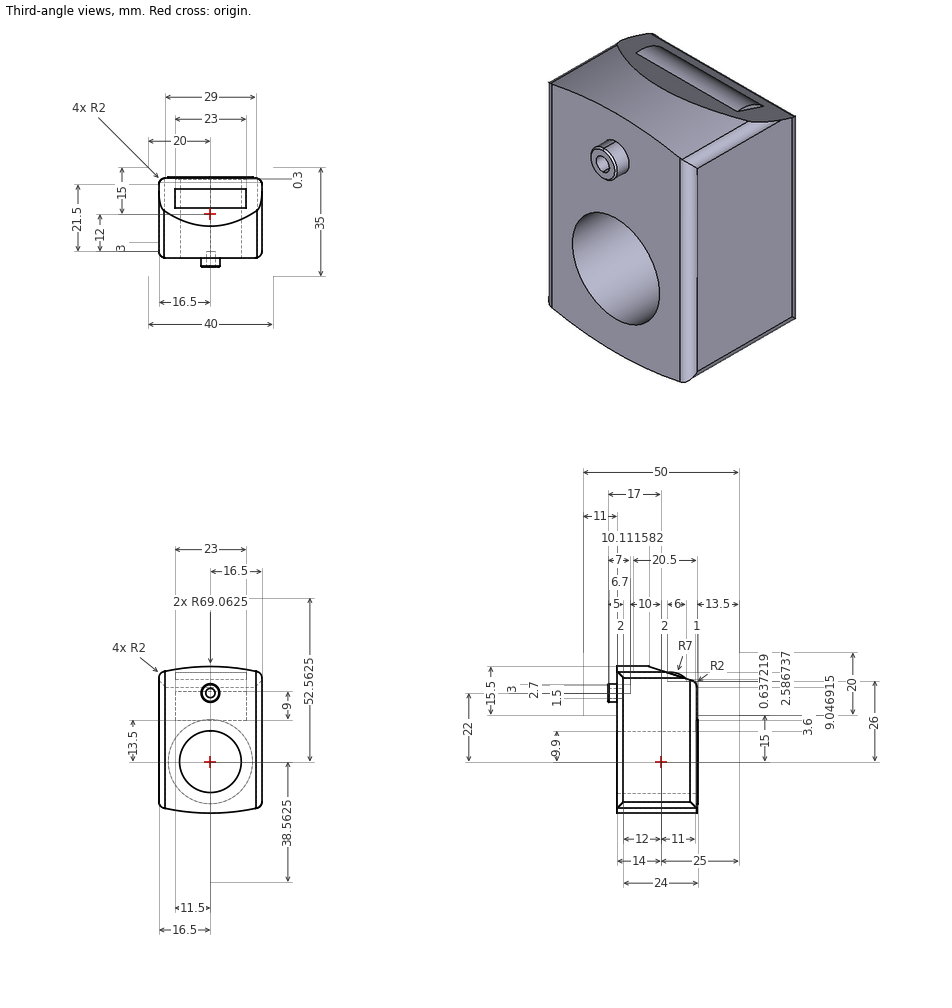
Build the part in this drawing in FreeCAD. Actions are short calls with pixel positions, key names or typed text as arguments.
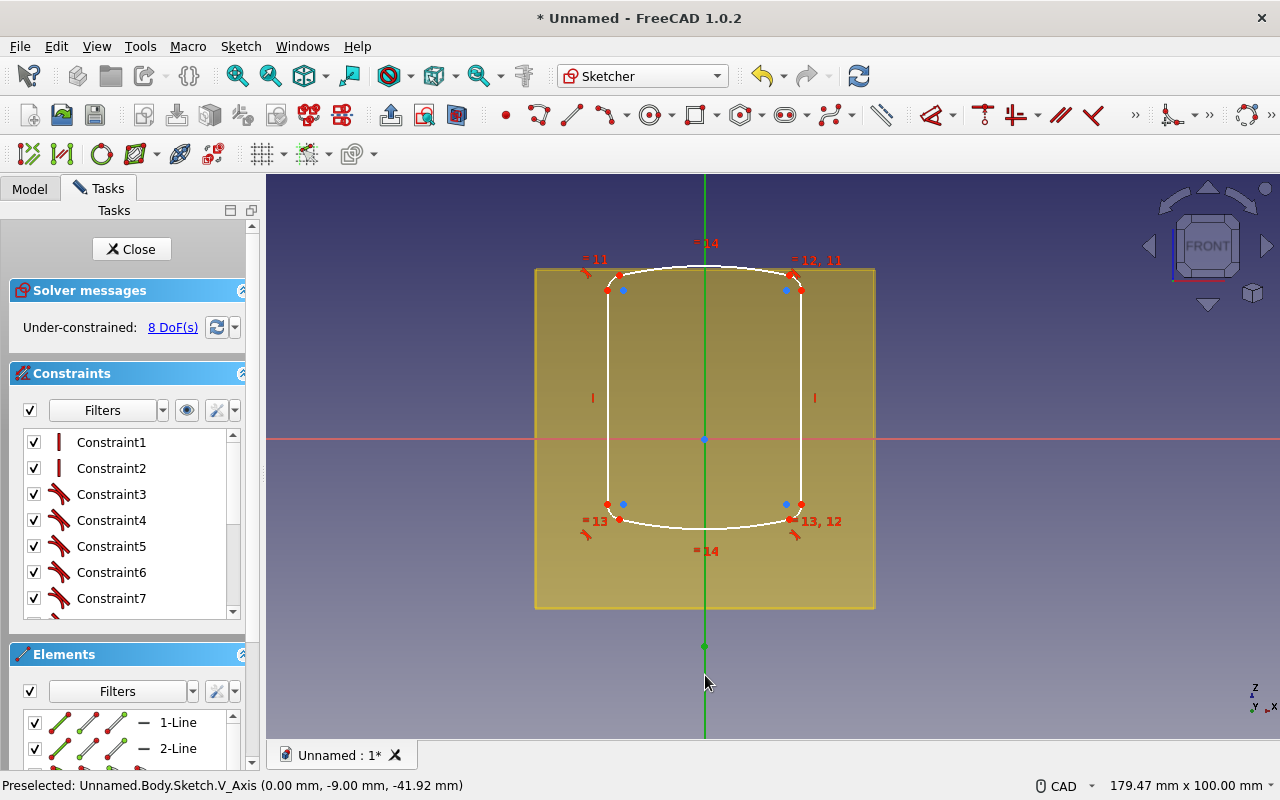
click(983, 116)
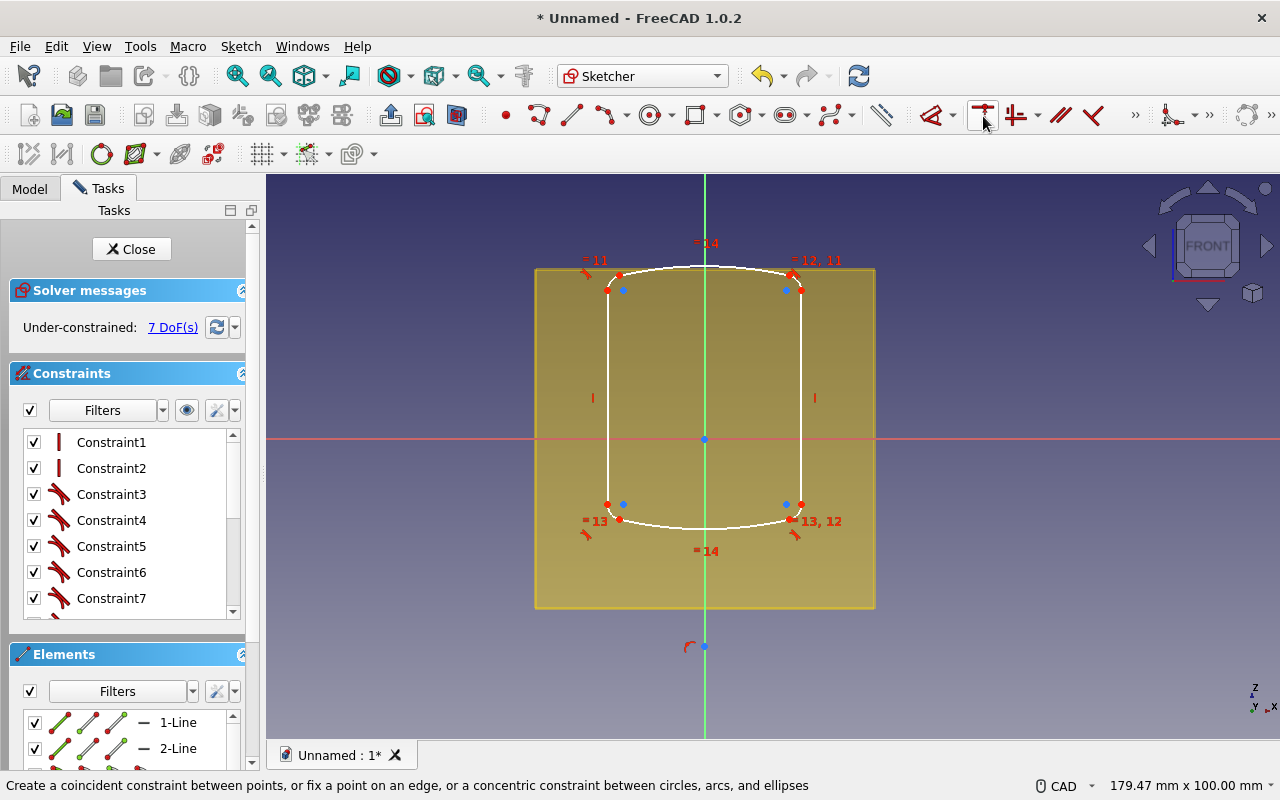
scroll(705, 284, up, 2)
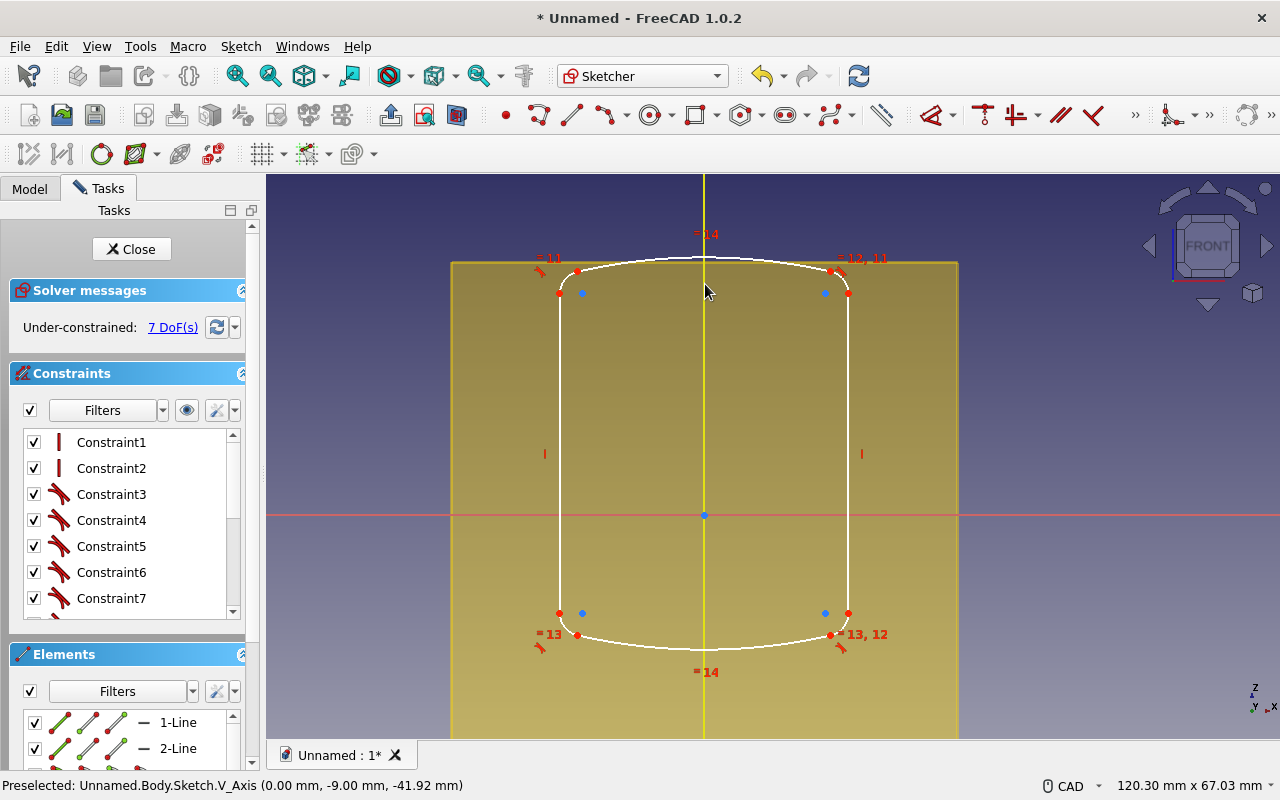
scroll(705, 635, down, 2)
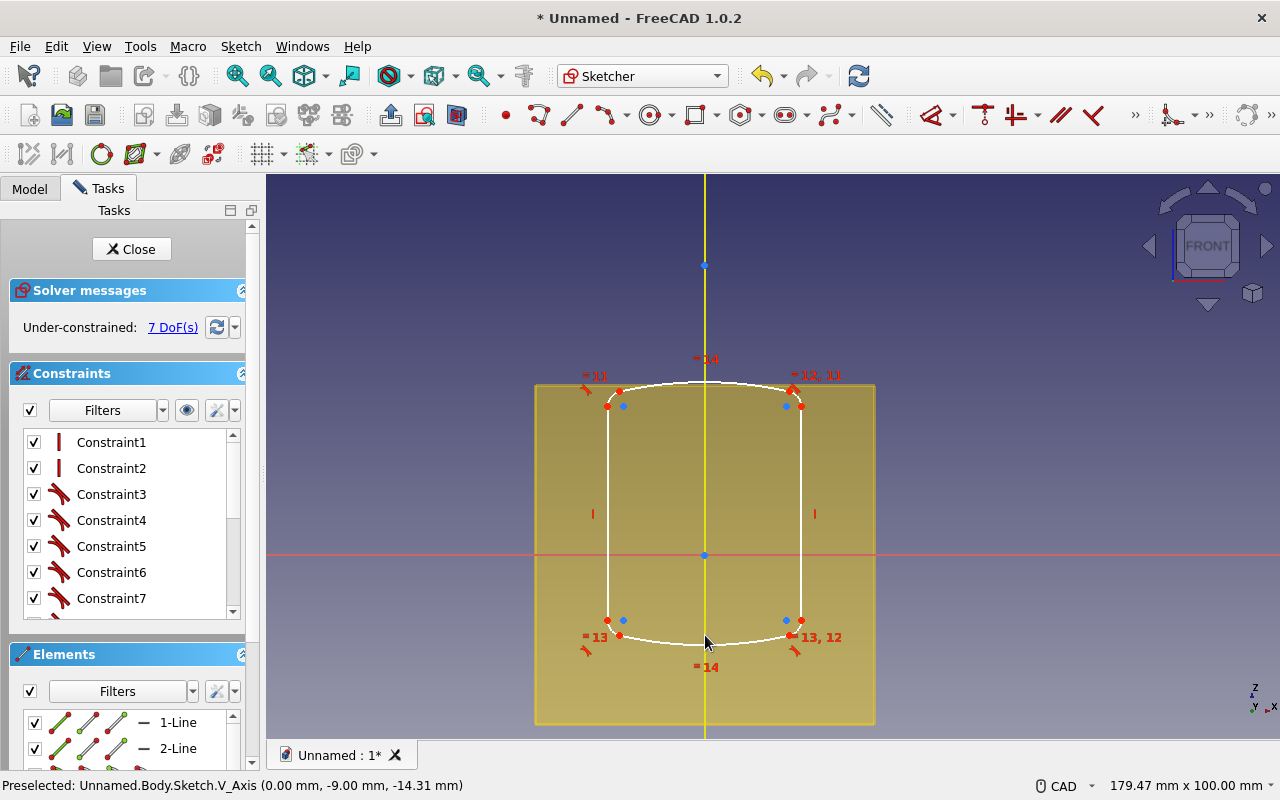
click(705, 265)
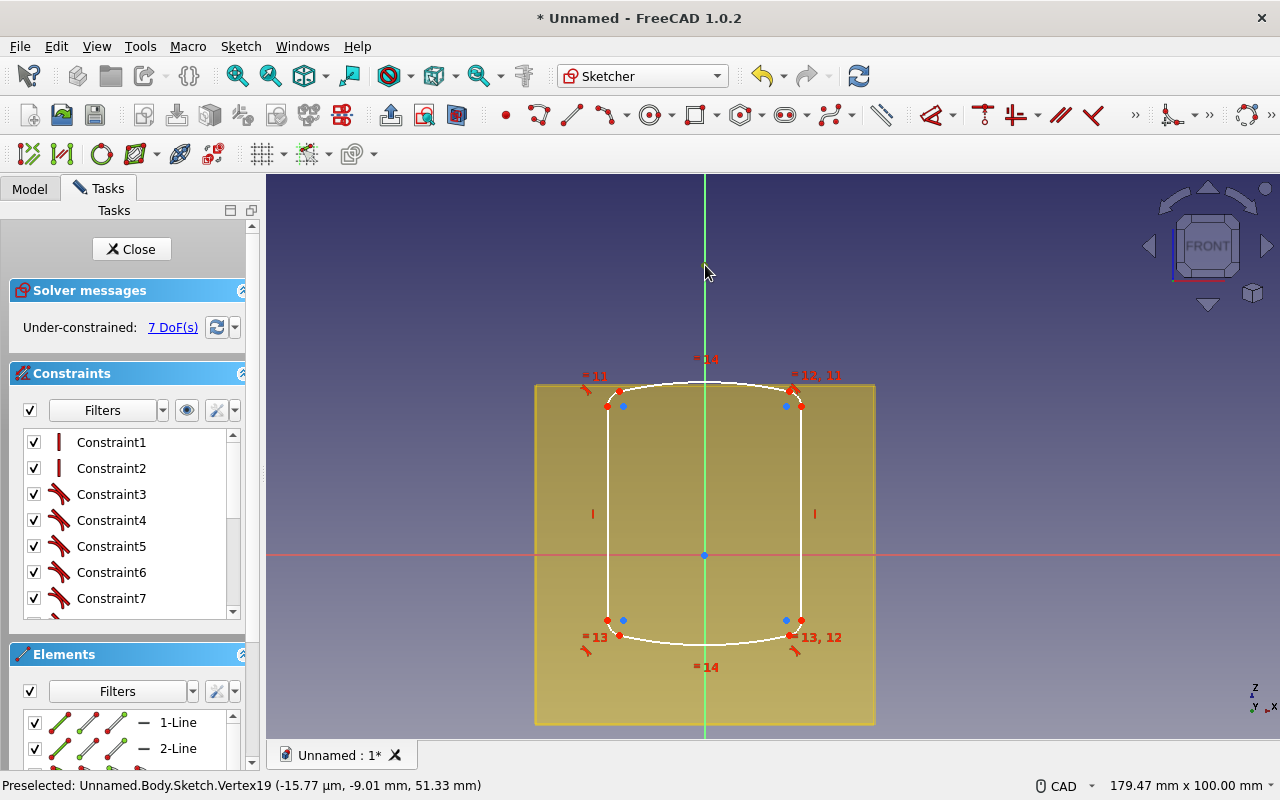
click(705, 602)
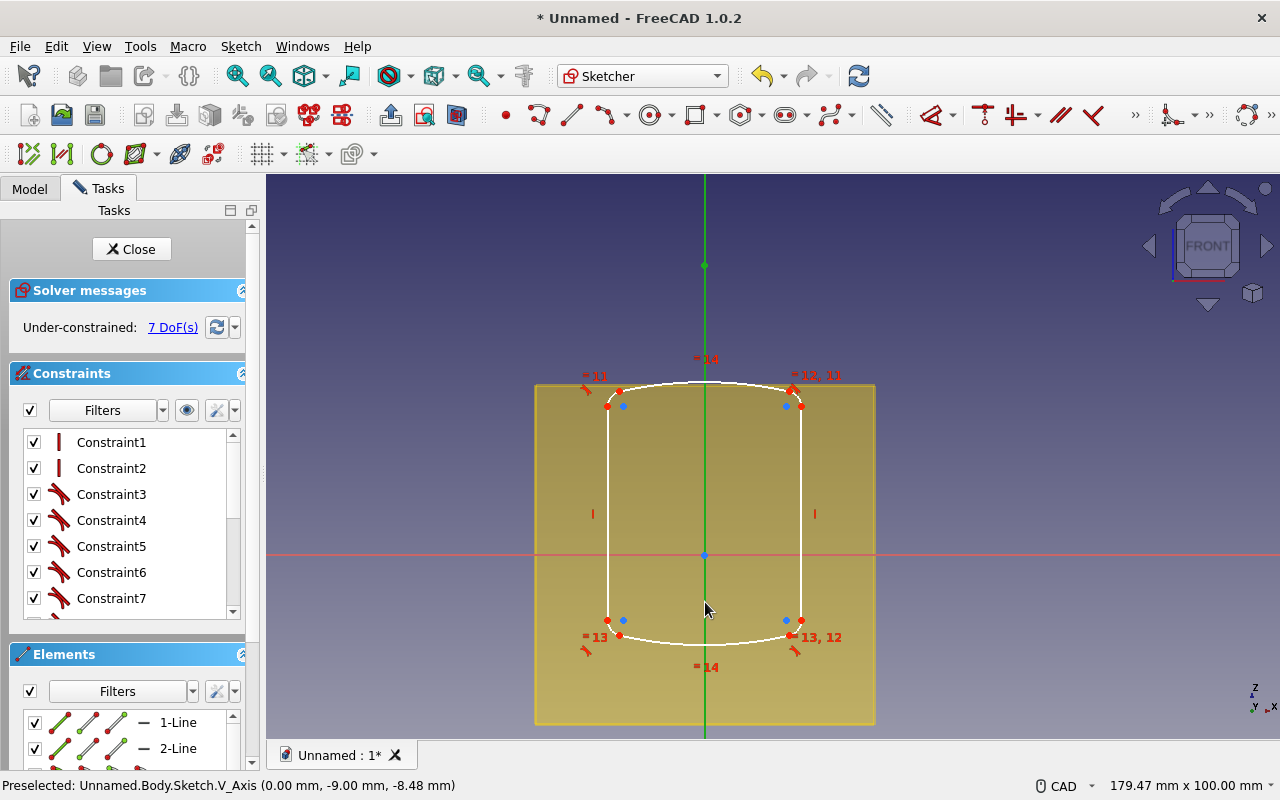
click(983, 116)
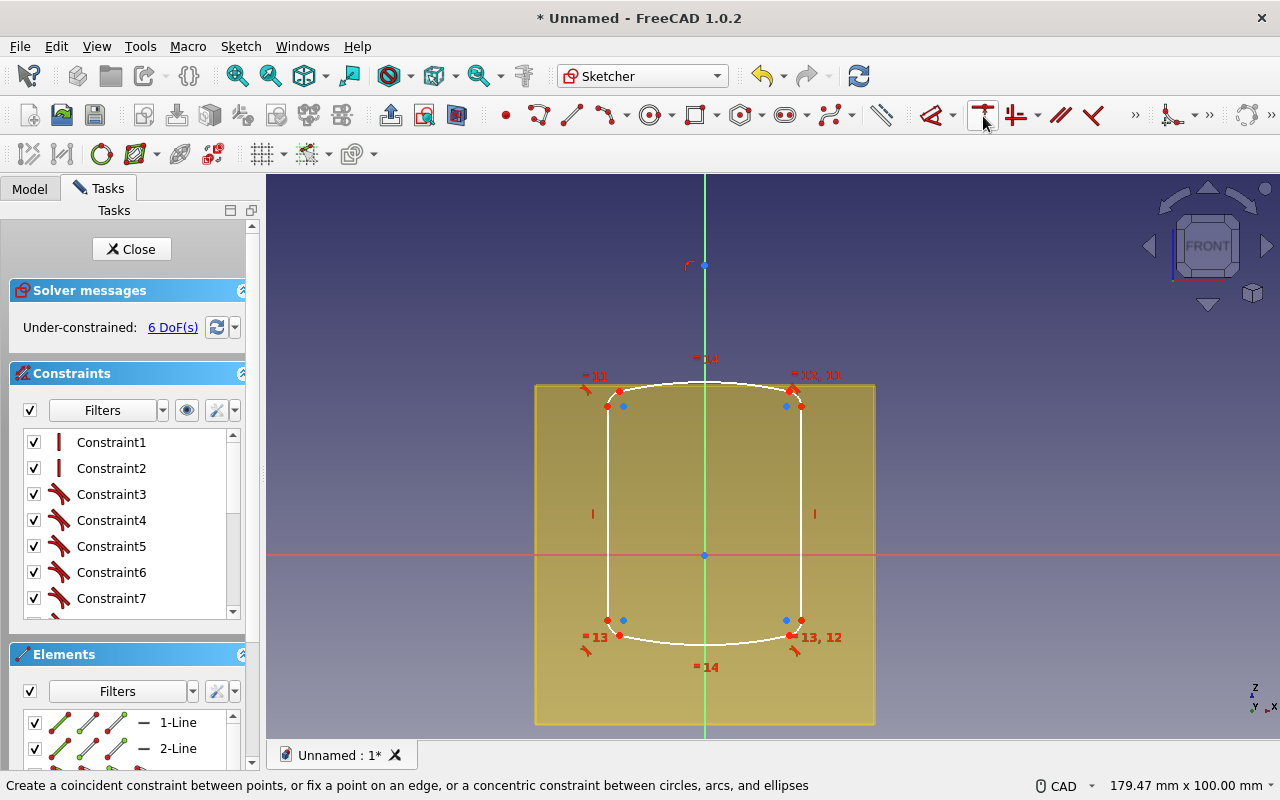
scroll(611, 397, up, 7)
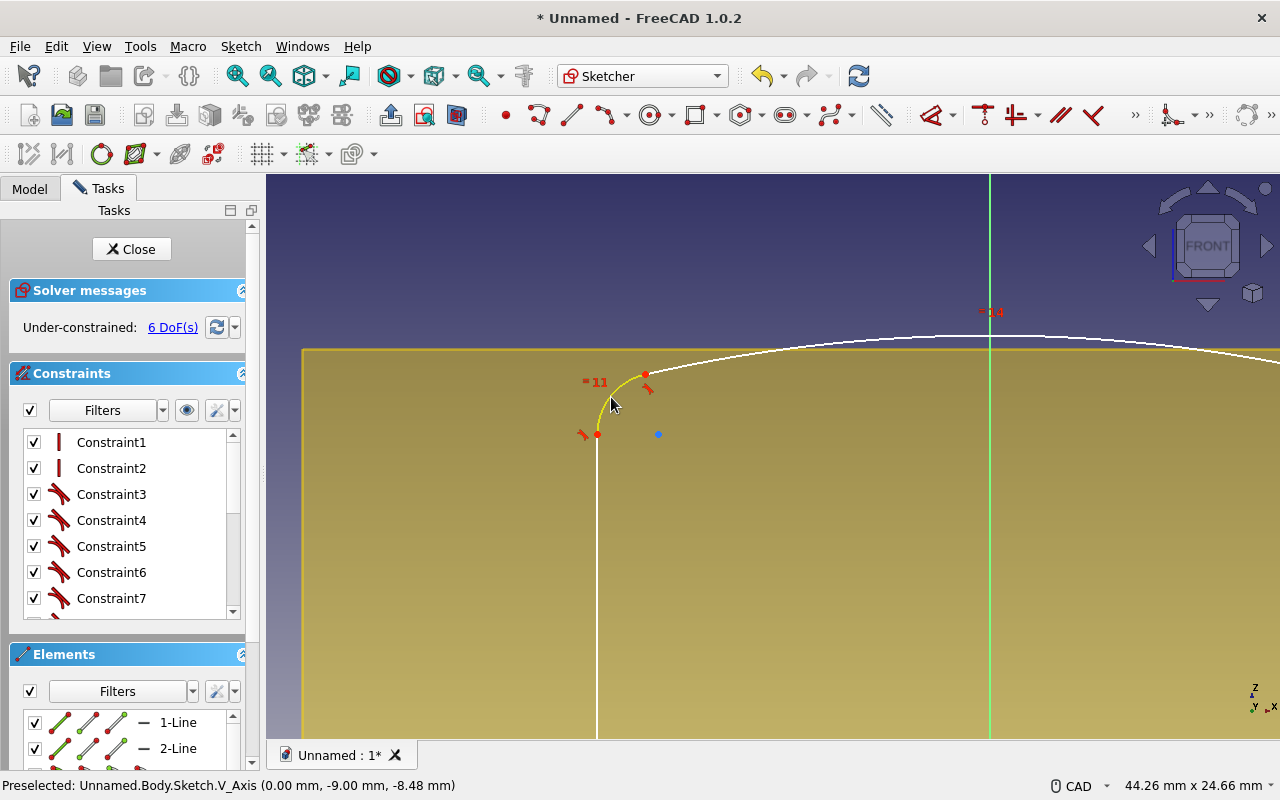
click(611, 396)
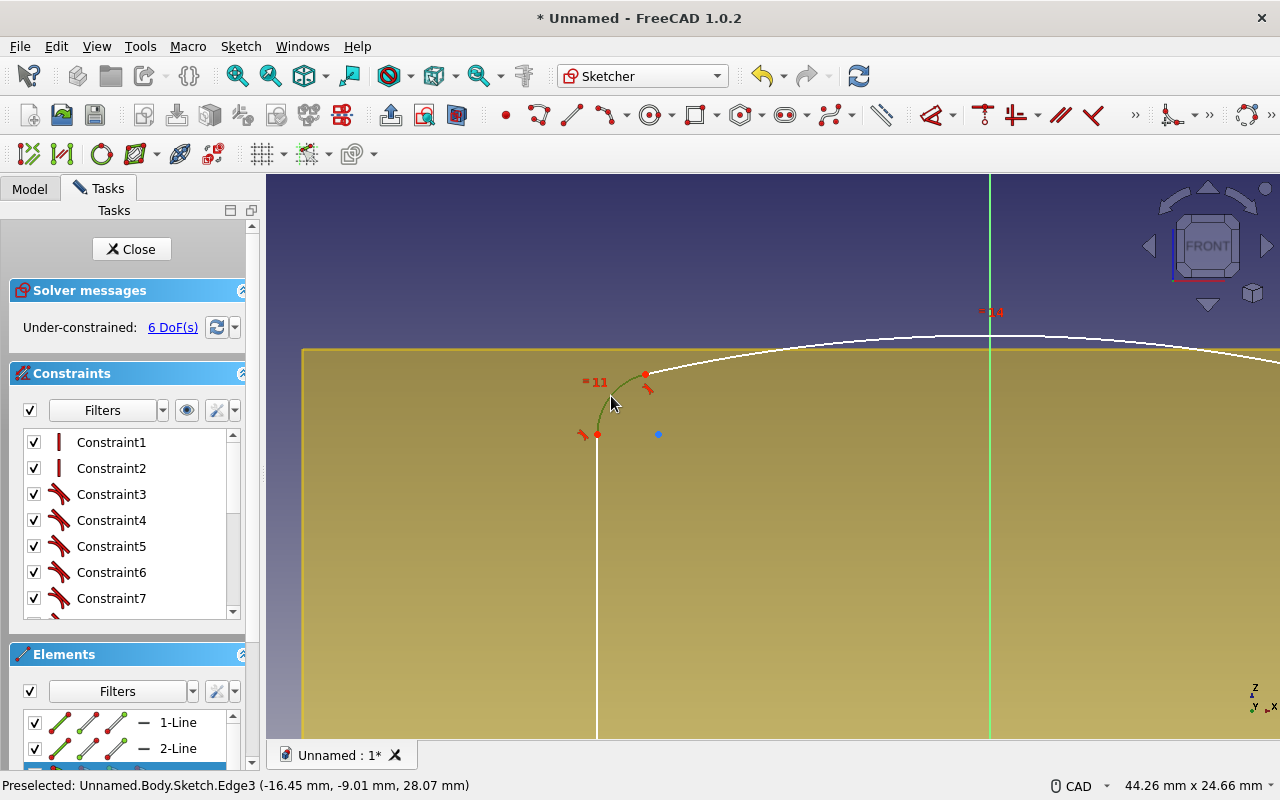
click(952, 116)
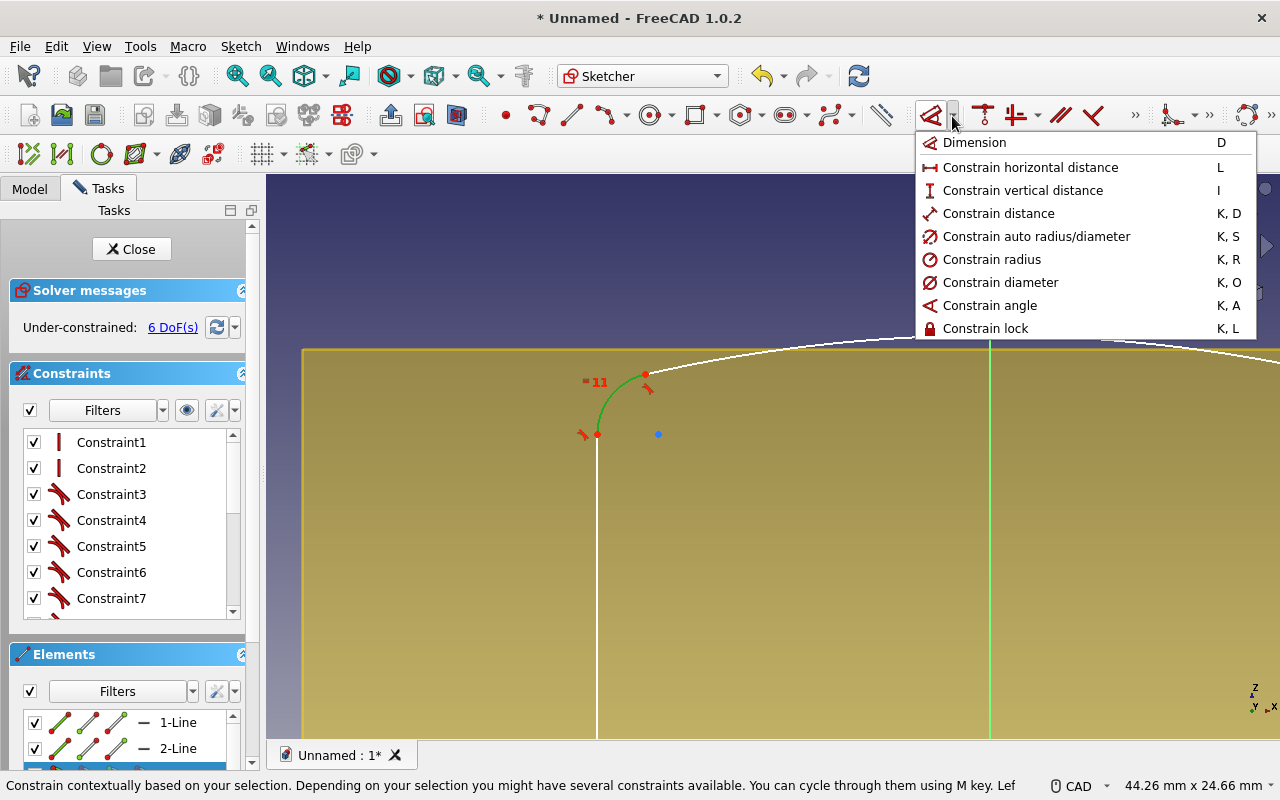
click(1086, 260)